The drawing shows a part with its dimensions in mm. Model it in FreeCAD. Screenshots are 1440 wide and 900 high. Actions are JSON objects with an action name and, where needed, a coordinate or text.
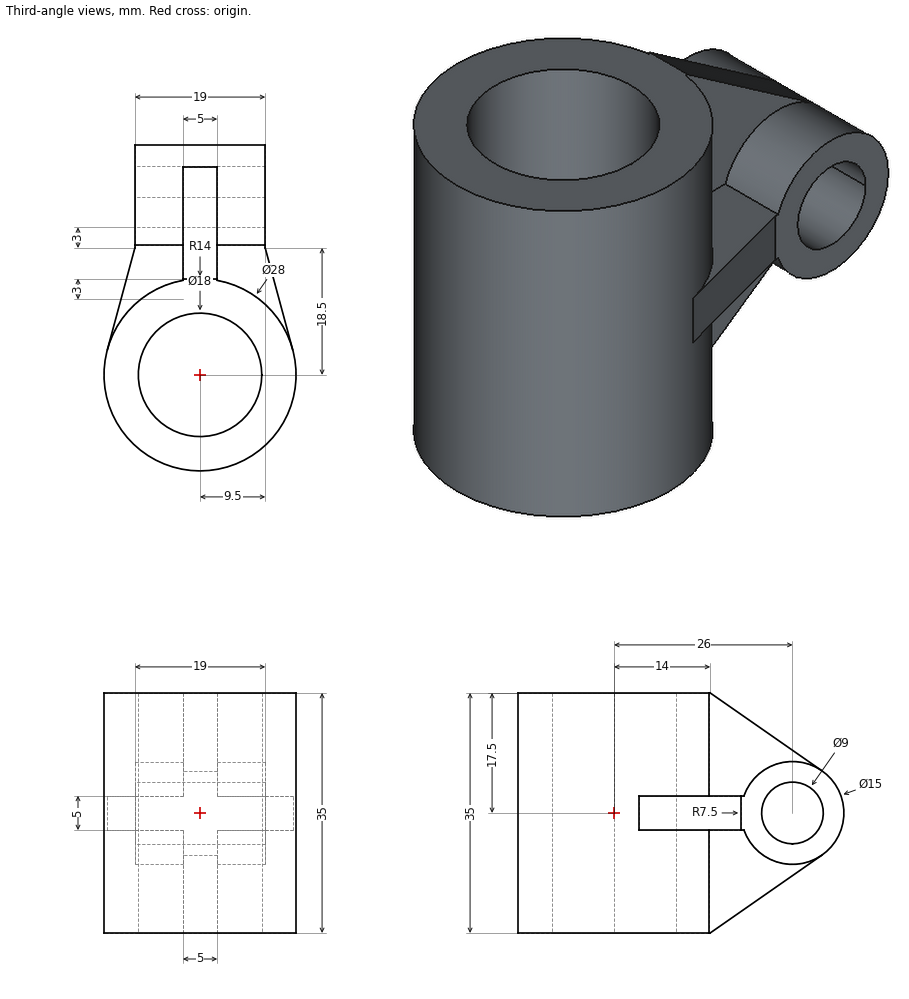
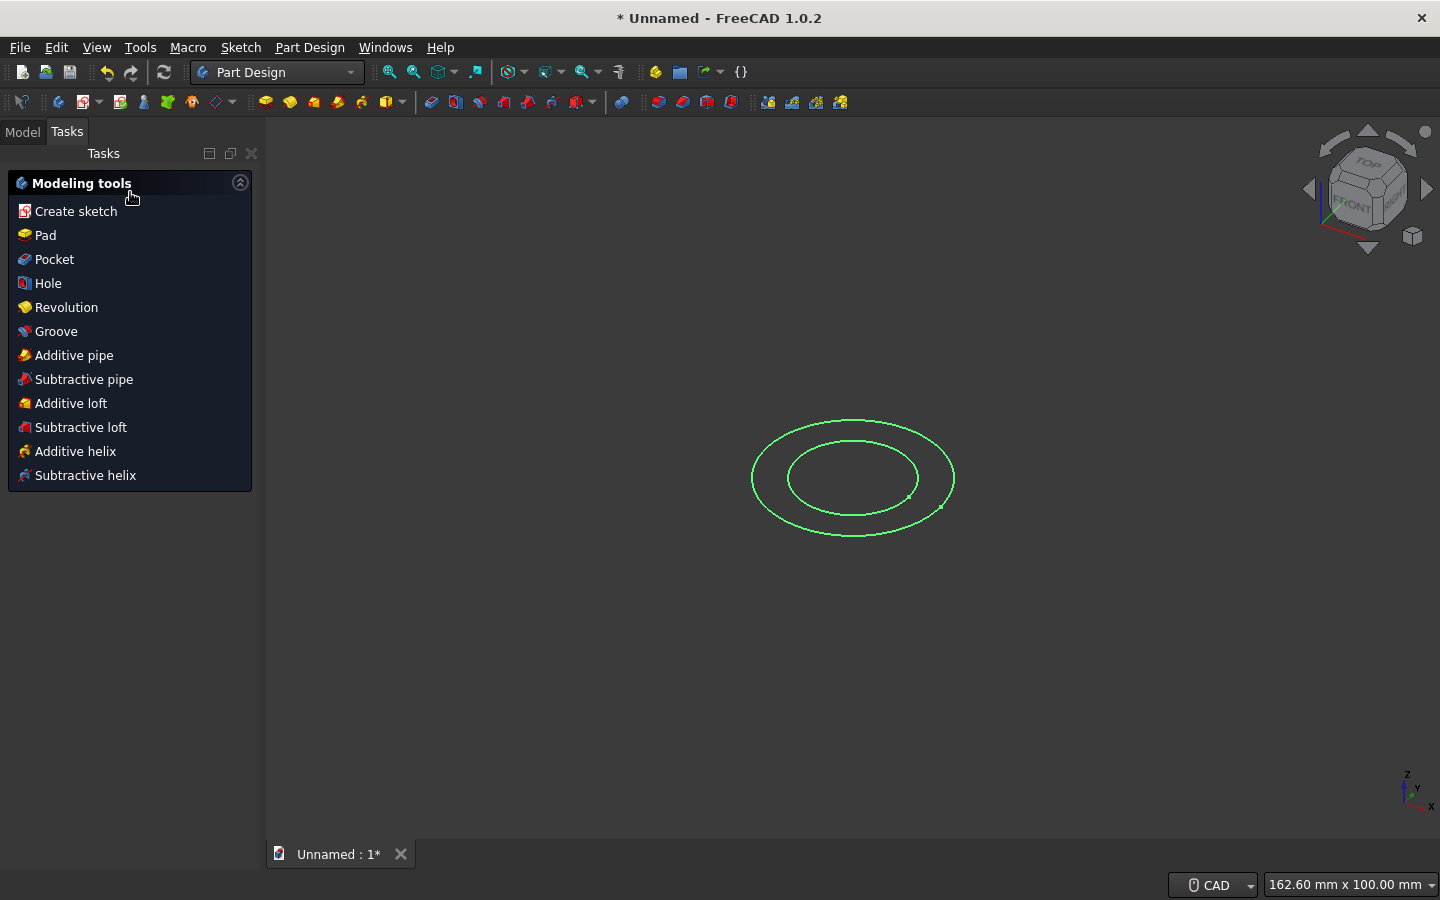
{"action": "left_click", "coordinate": [266, 102]}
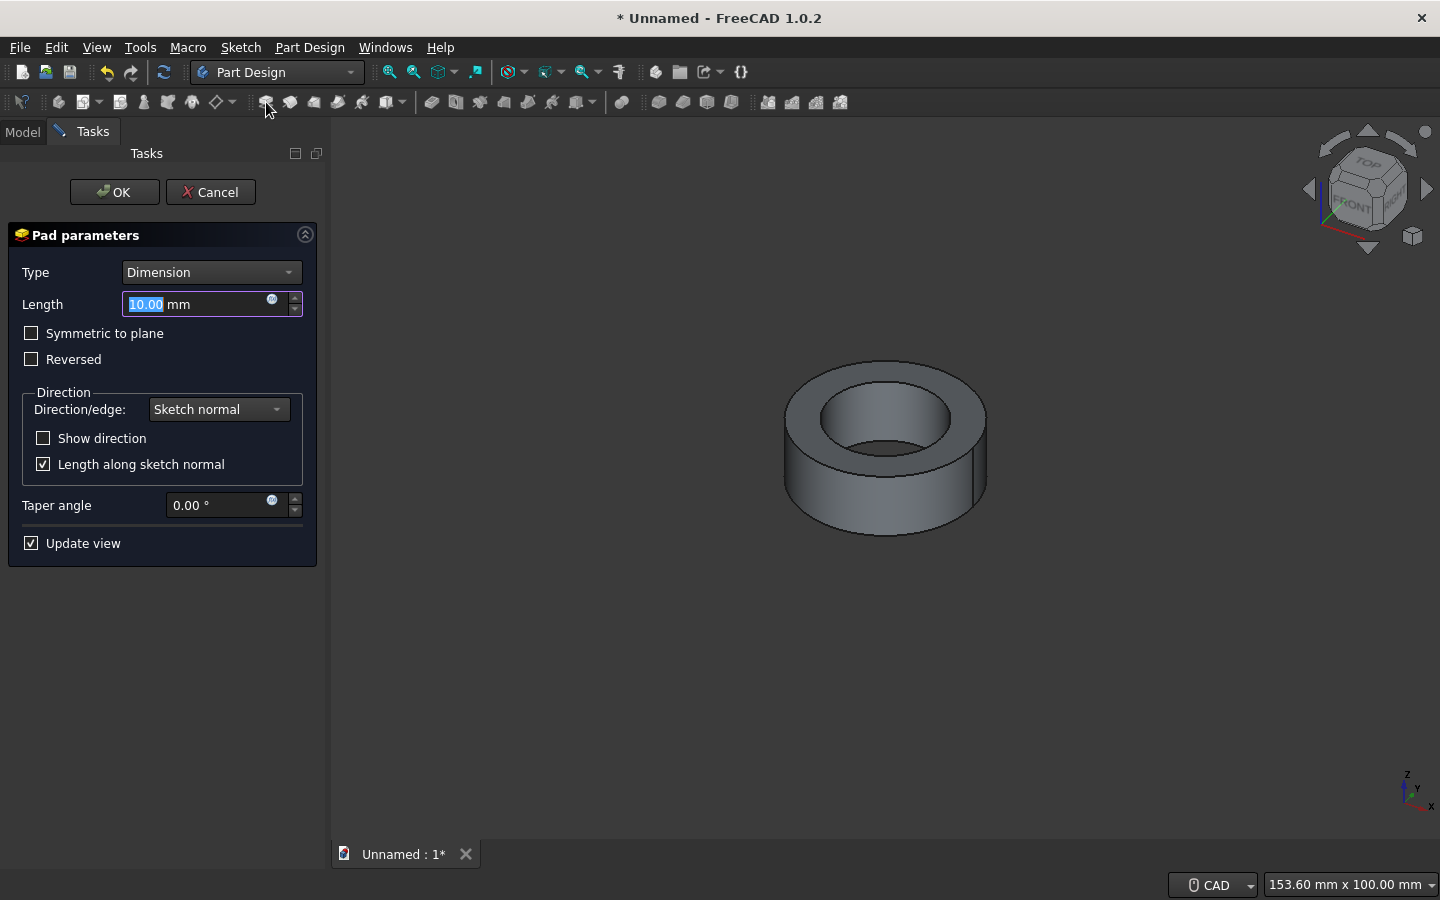
{"action": "type", "text": "35"}
{"action": "key", "text": "Tab"}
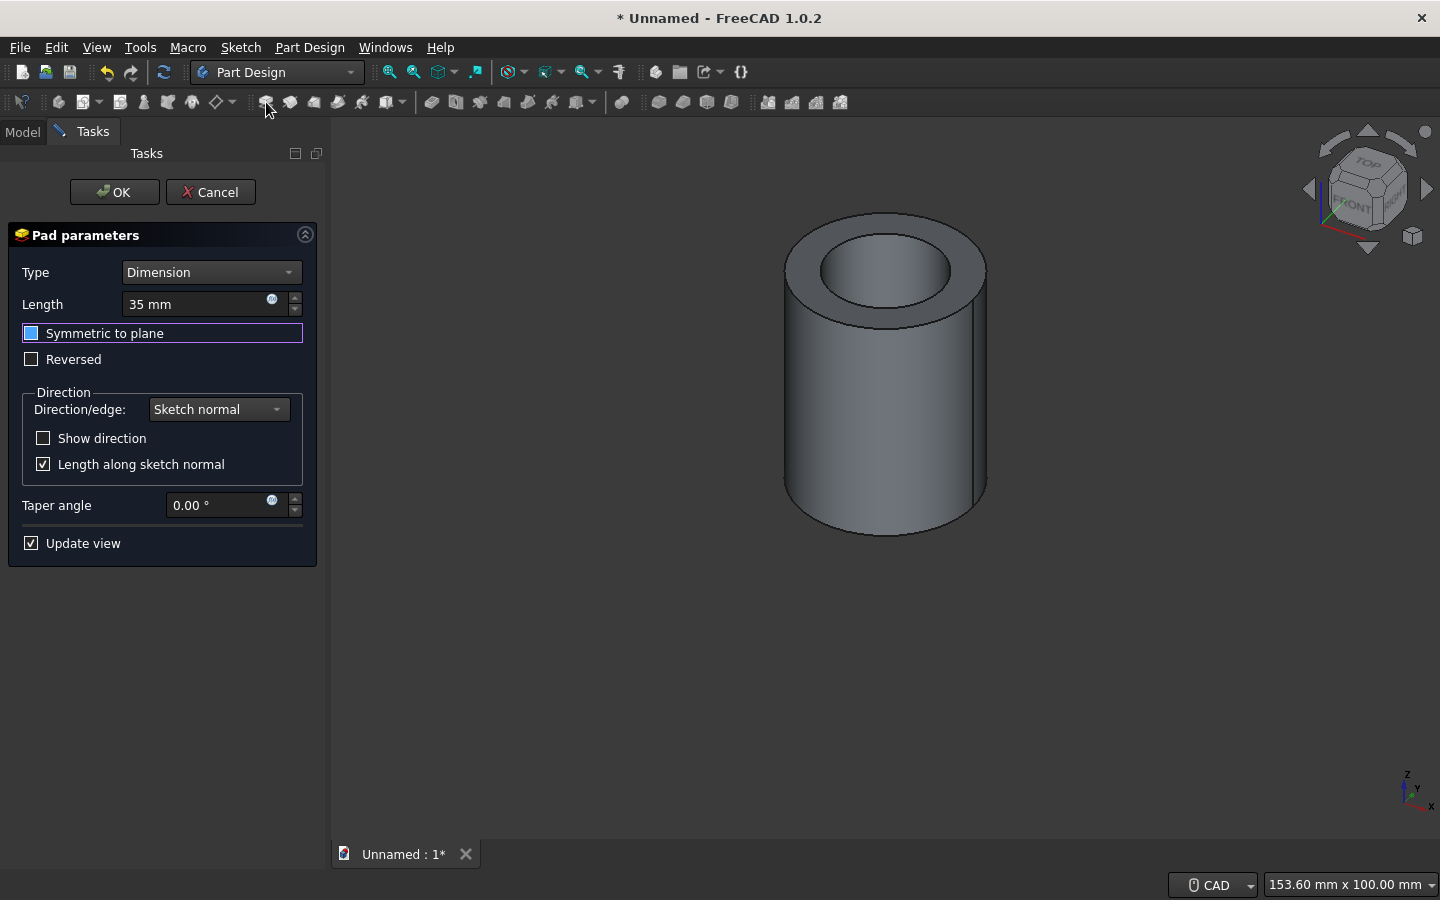
{"action": "left_click", "coordinate": [30, 333]}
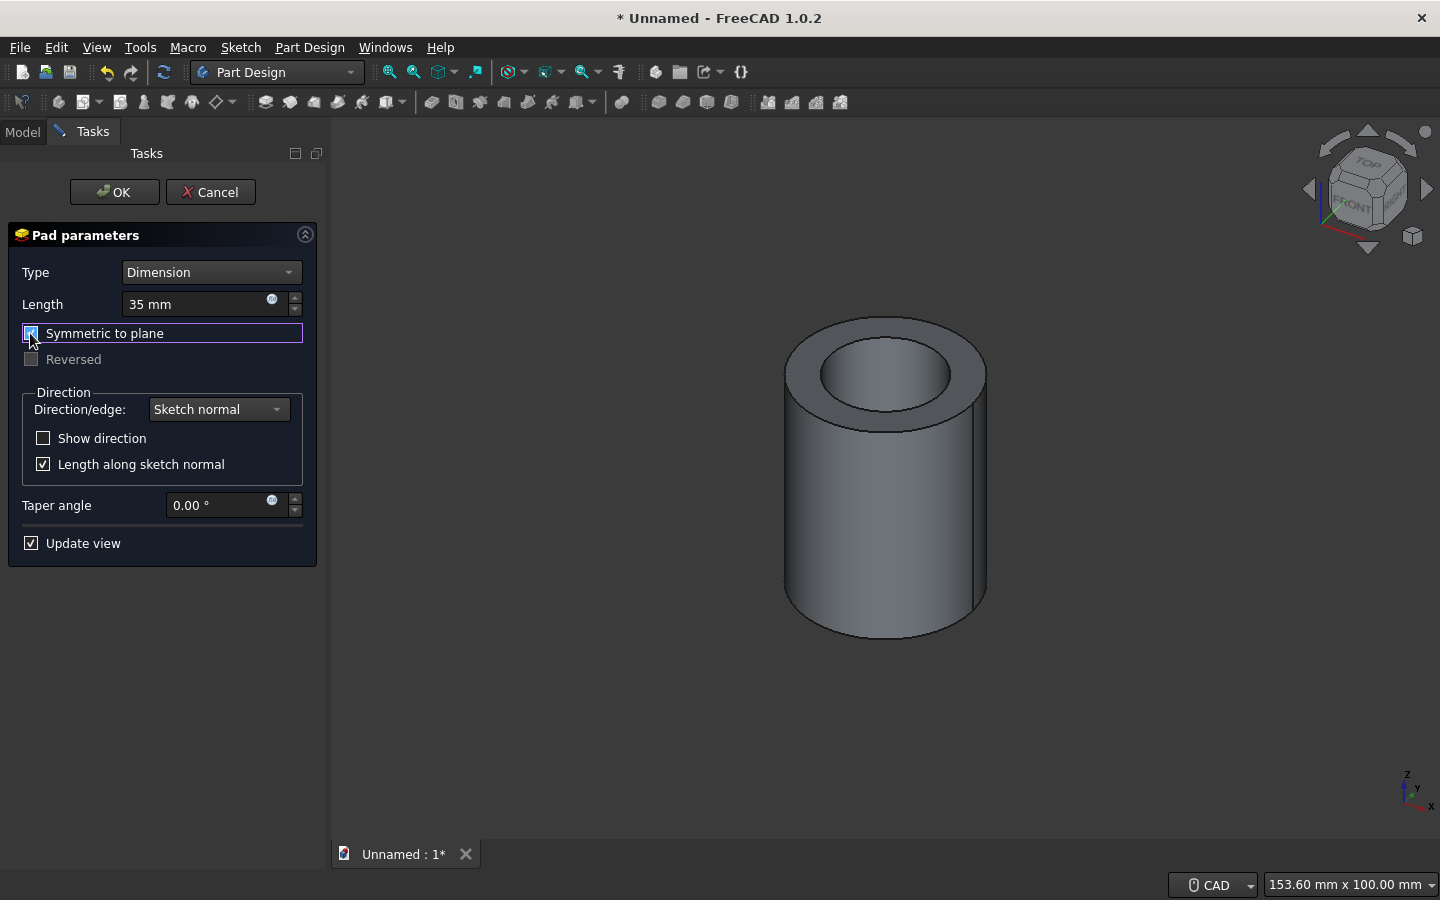
{"action": "left_click", "coordinate": [115, 192]}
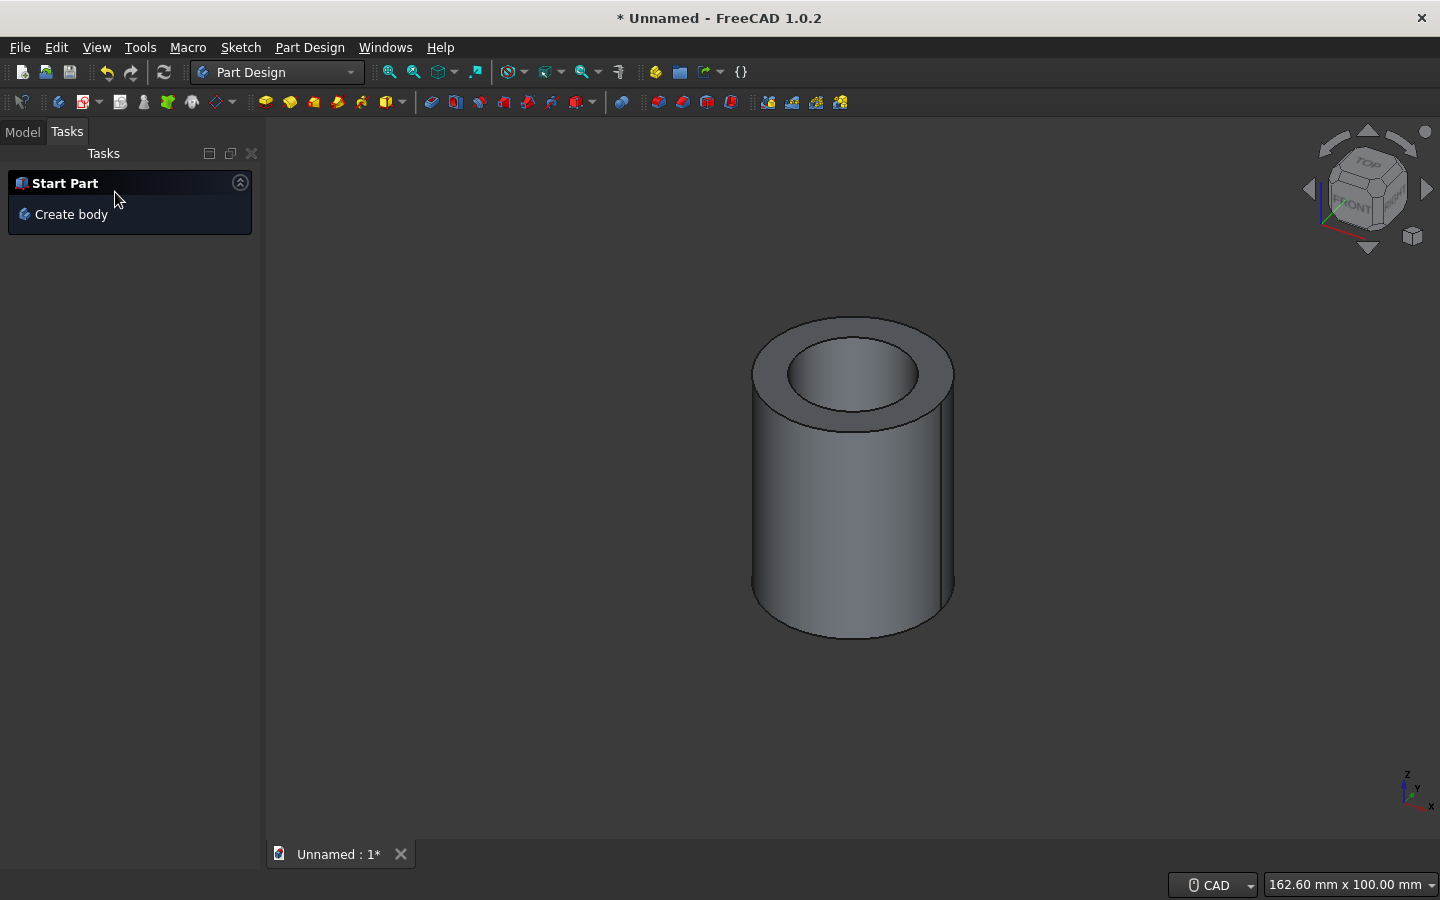
{"action": "left_click", "coordinate": [60, 102]}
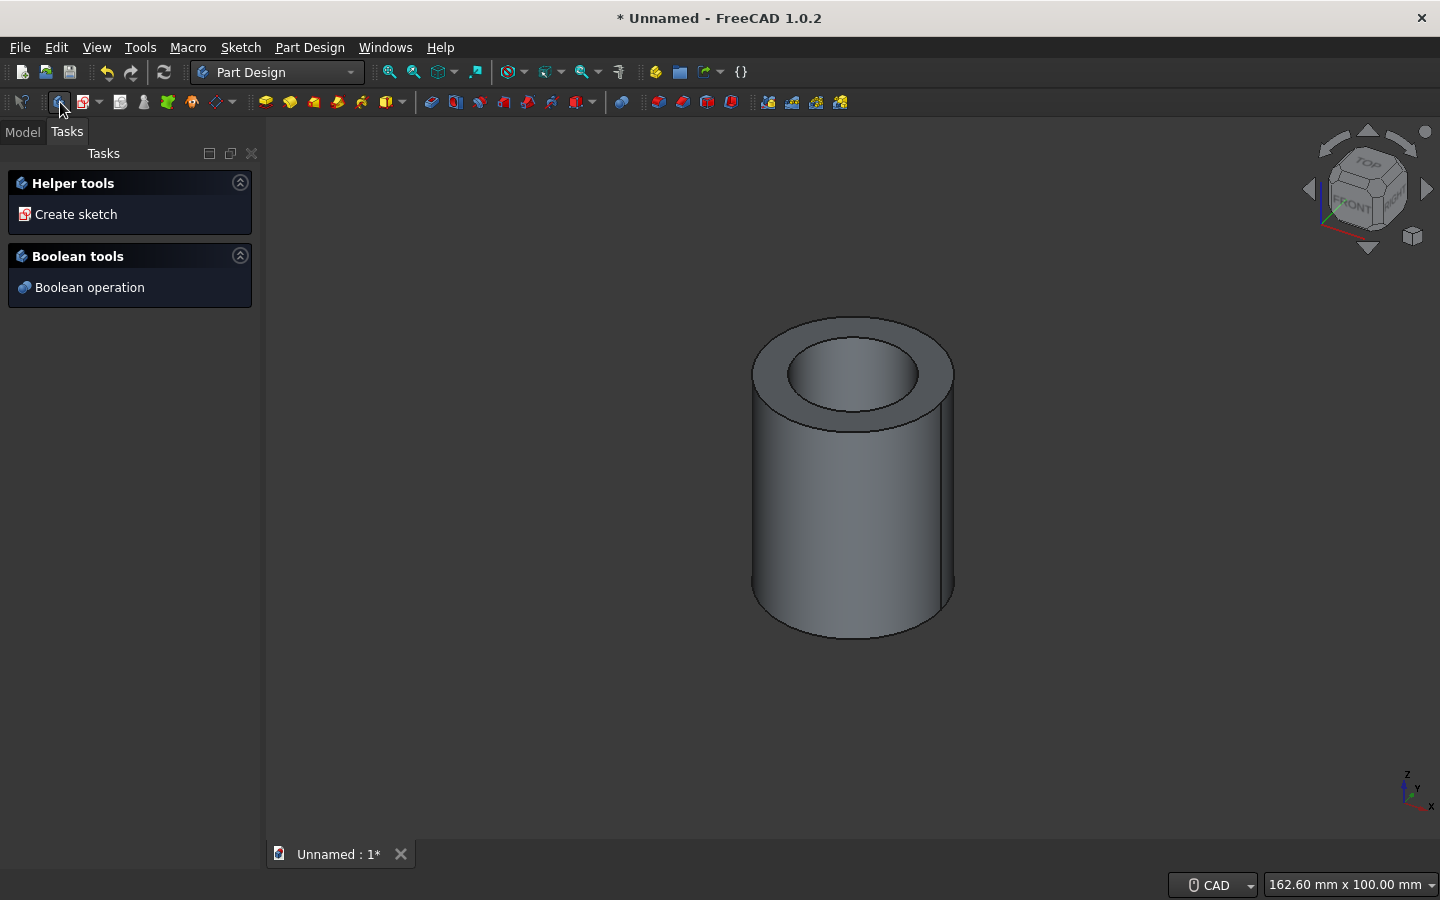
{"action": "left_click", "coordinate": [306, 799]}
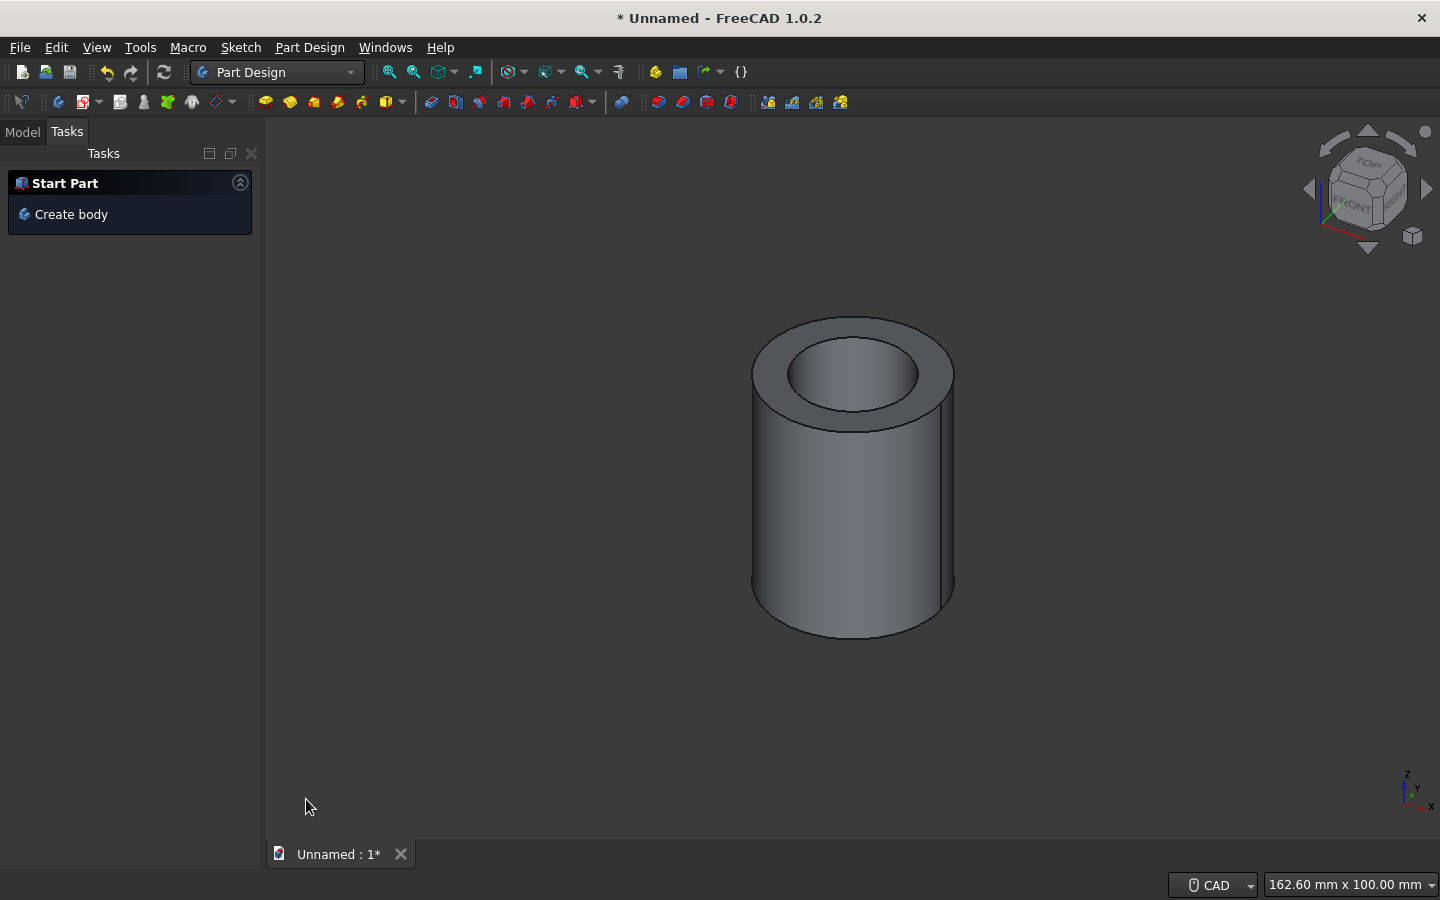
{"action": "left_click", "coordinate": [84, 102]}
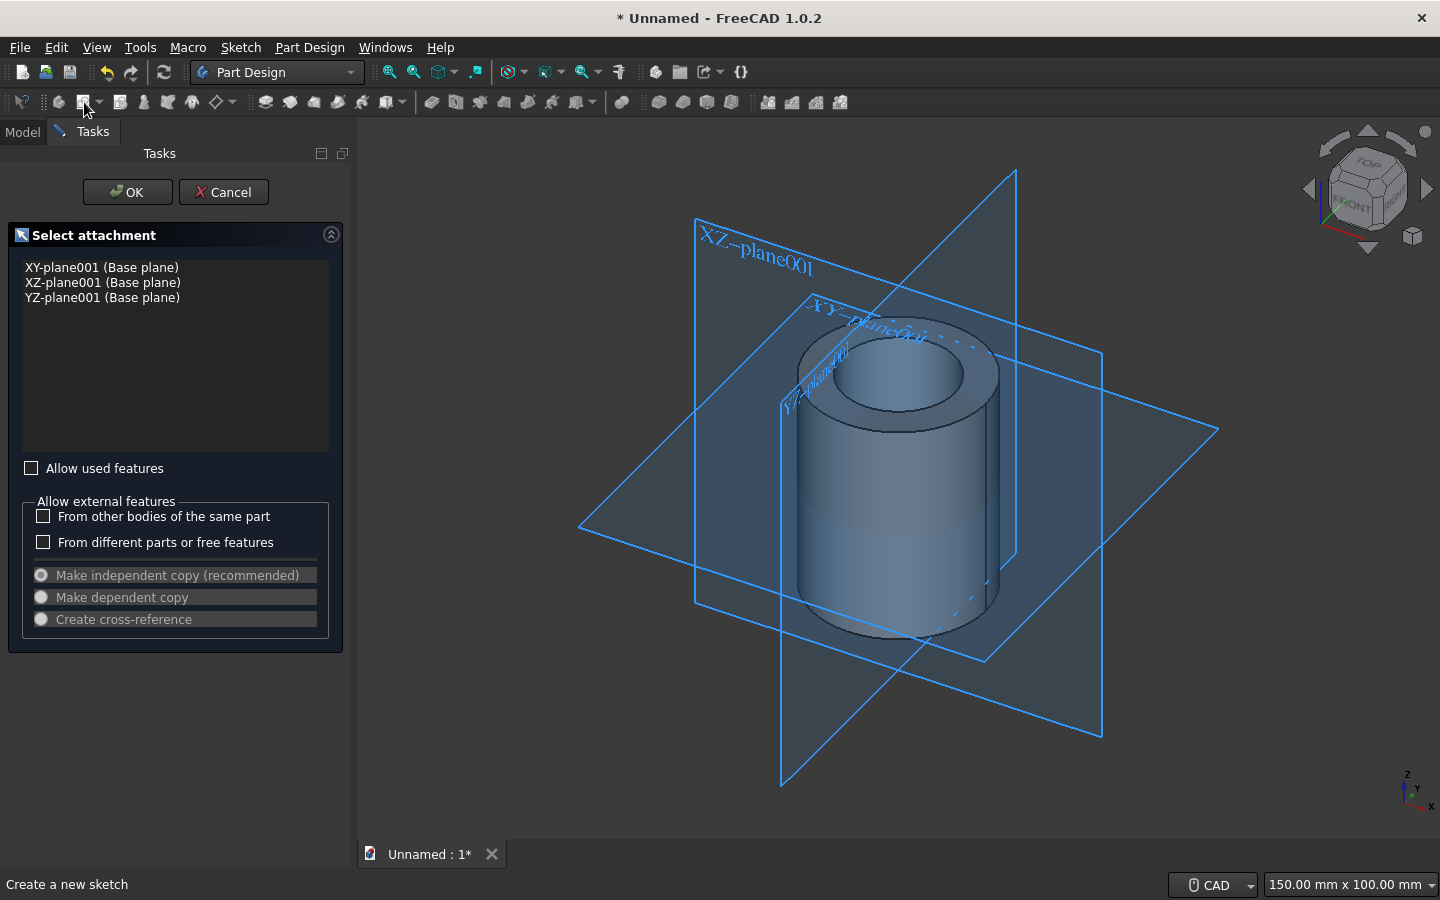
{"action": "left_click", "coordinate": [82, 298]}